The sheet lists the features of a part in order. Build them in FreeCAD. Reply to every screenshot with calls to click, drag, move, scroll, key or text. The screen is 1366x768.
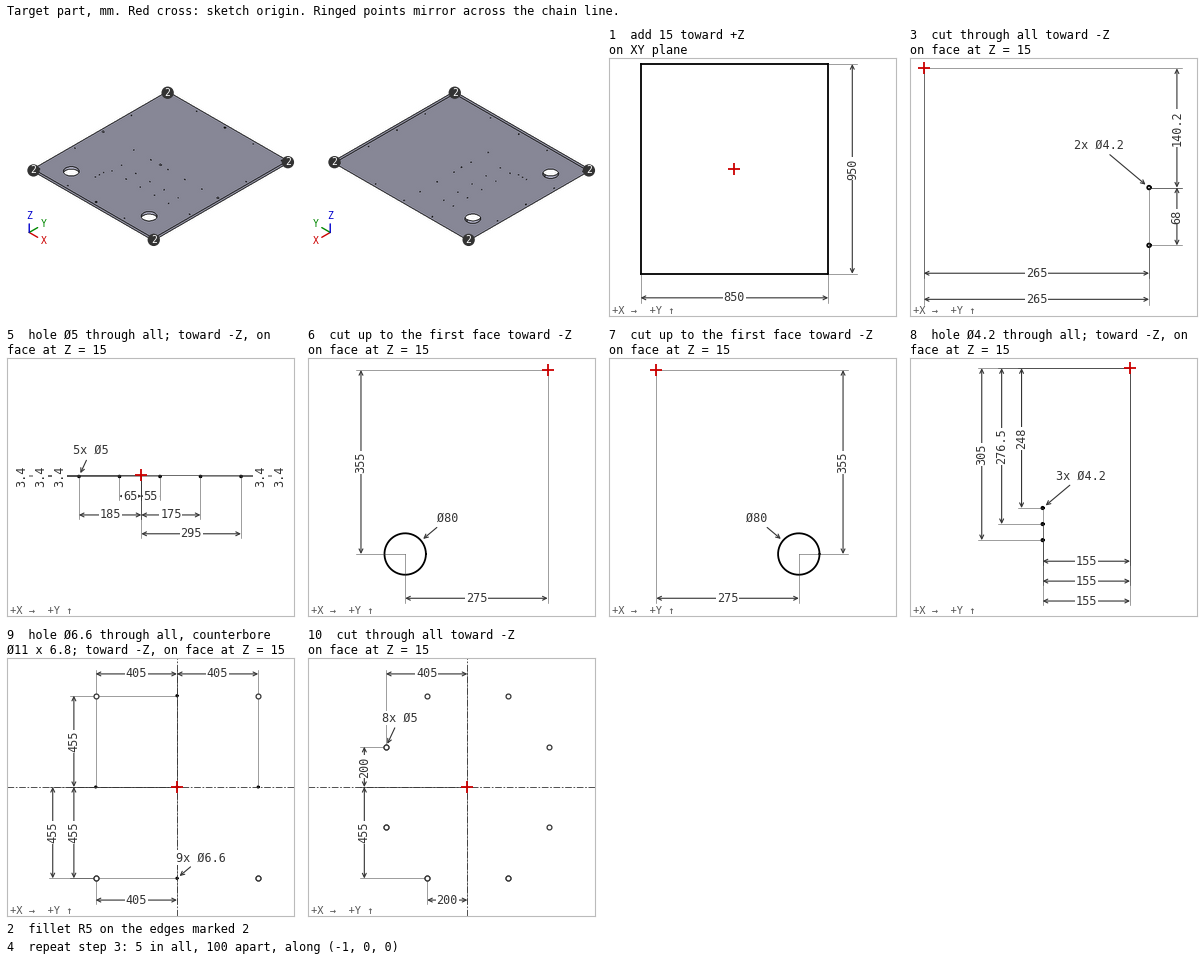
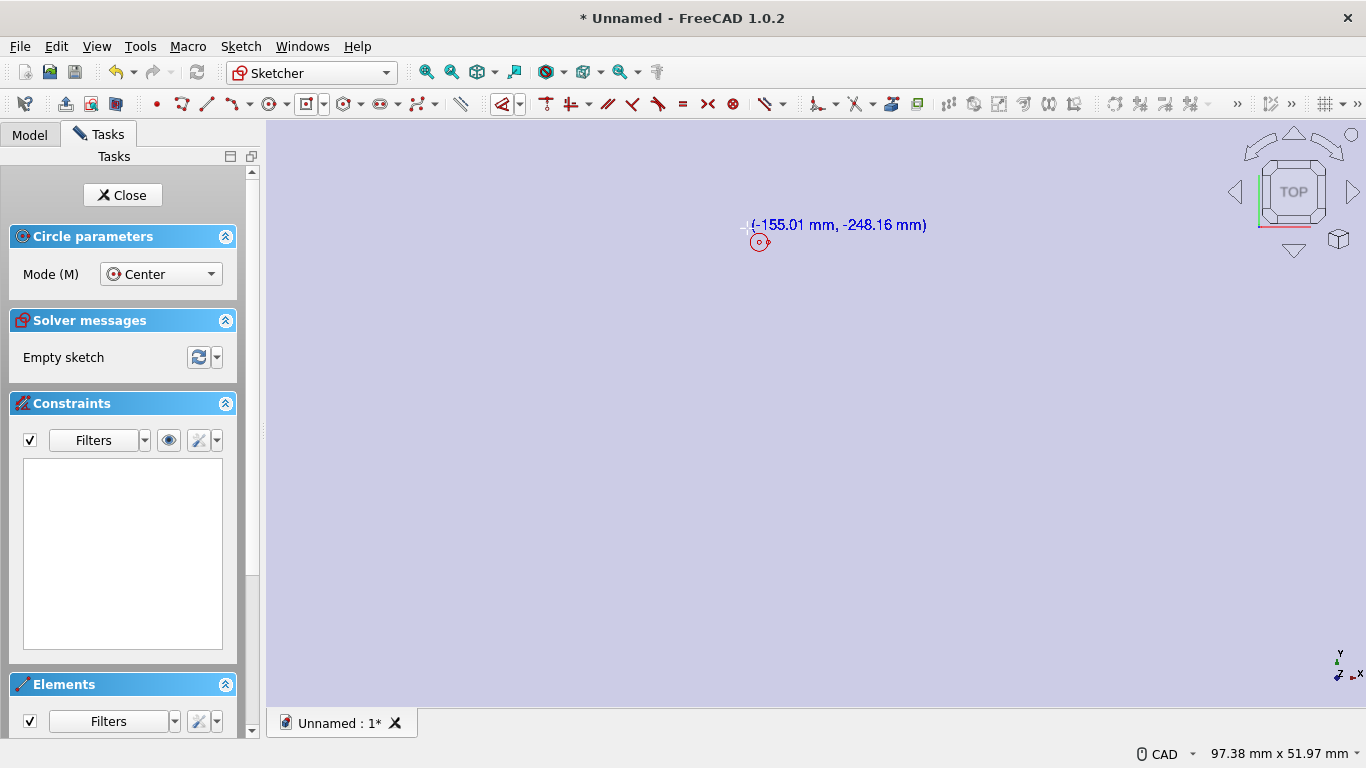
click(747, 228)
move(764, 211)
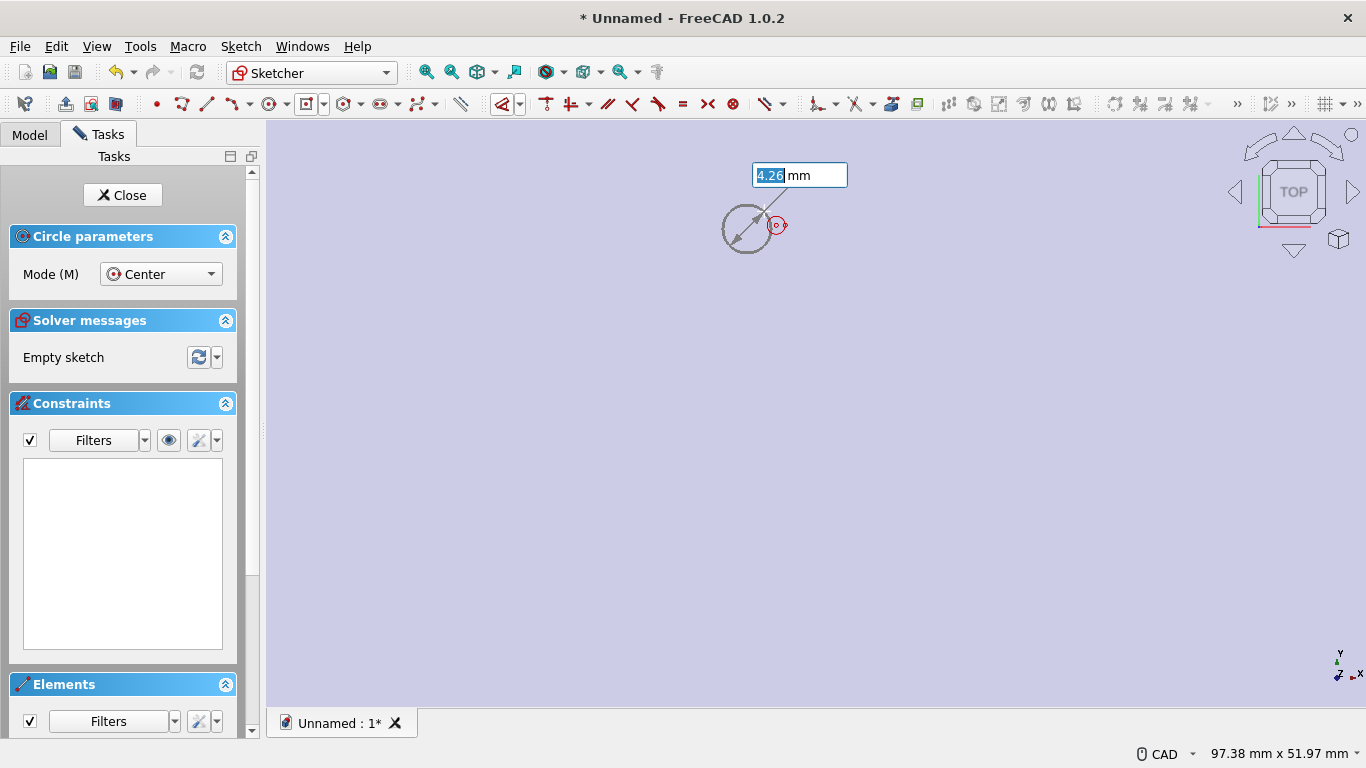
text(4.2)
key(Return)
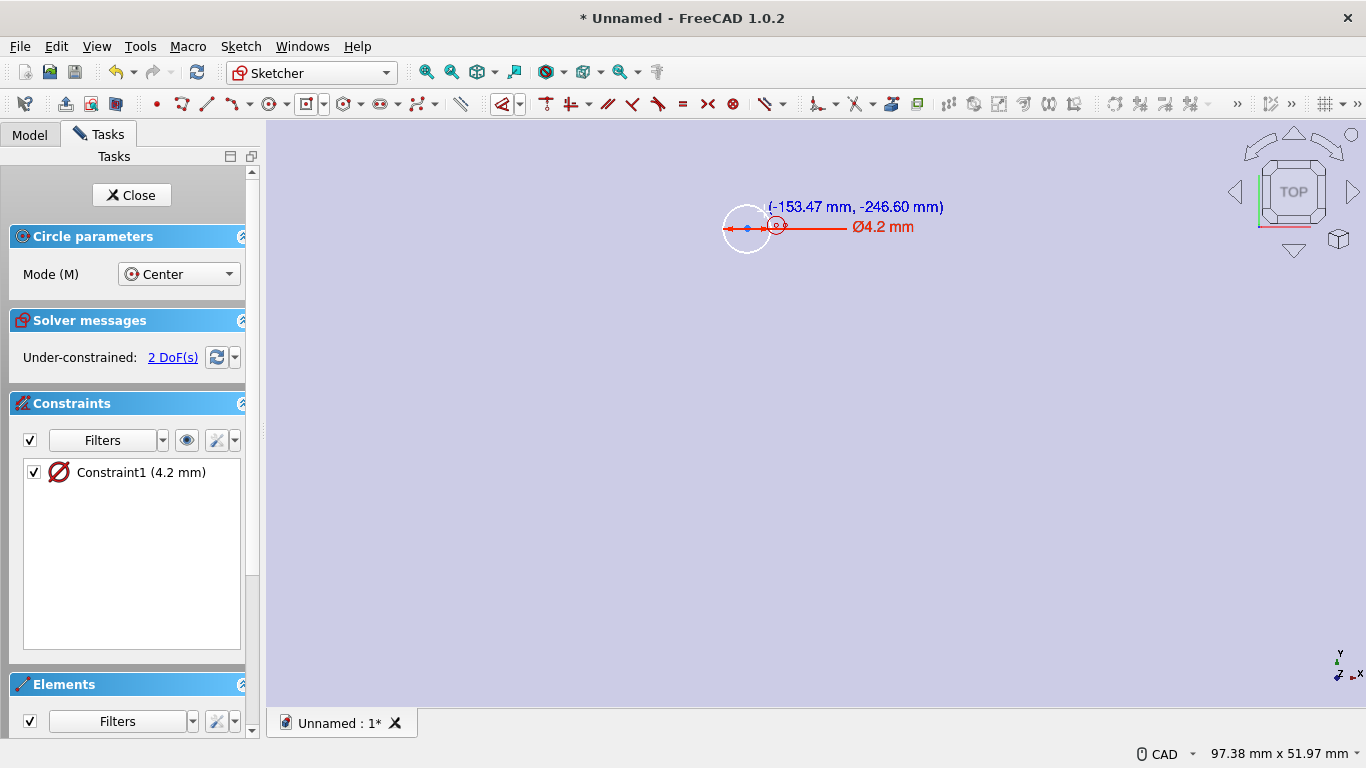
click(747, 550)
move(764, 533)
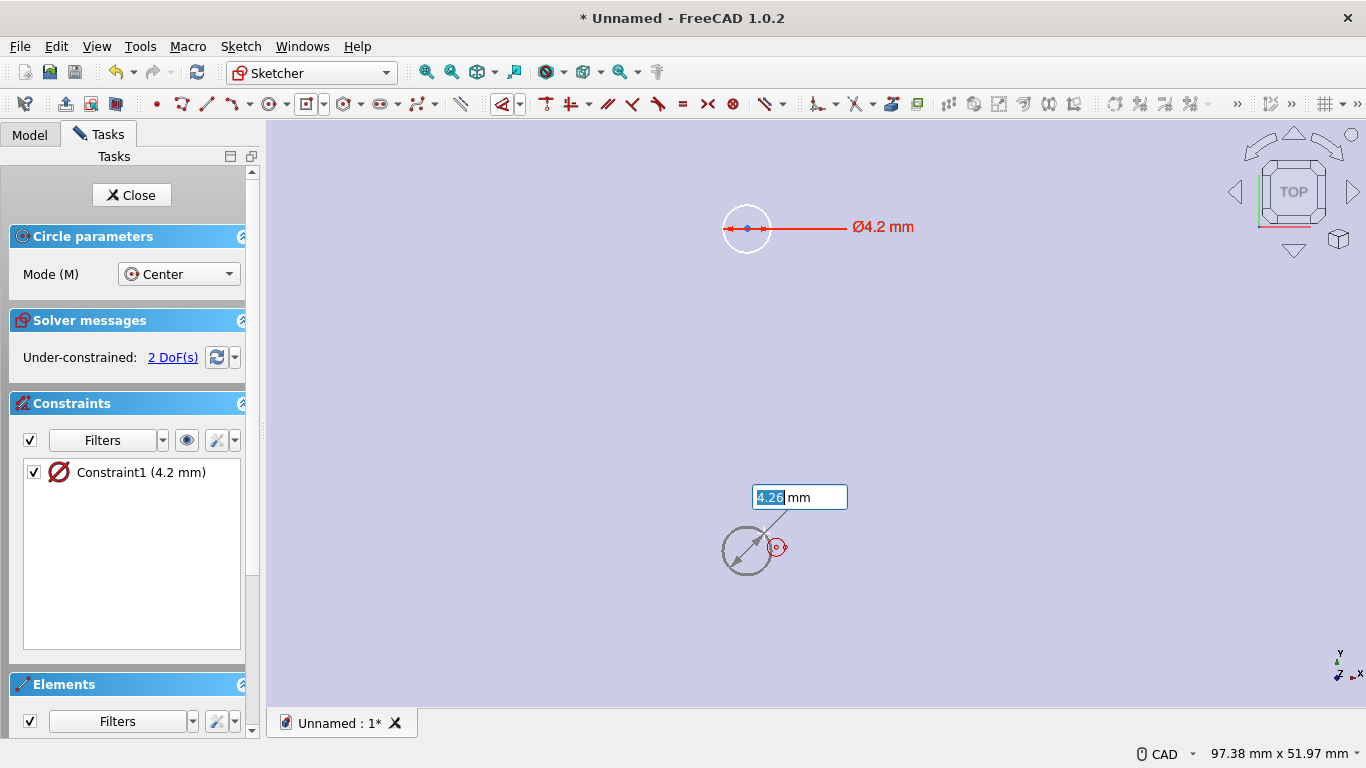
text(4.2)
key(Return)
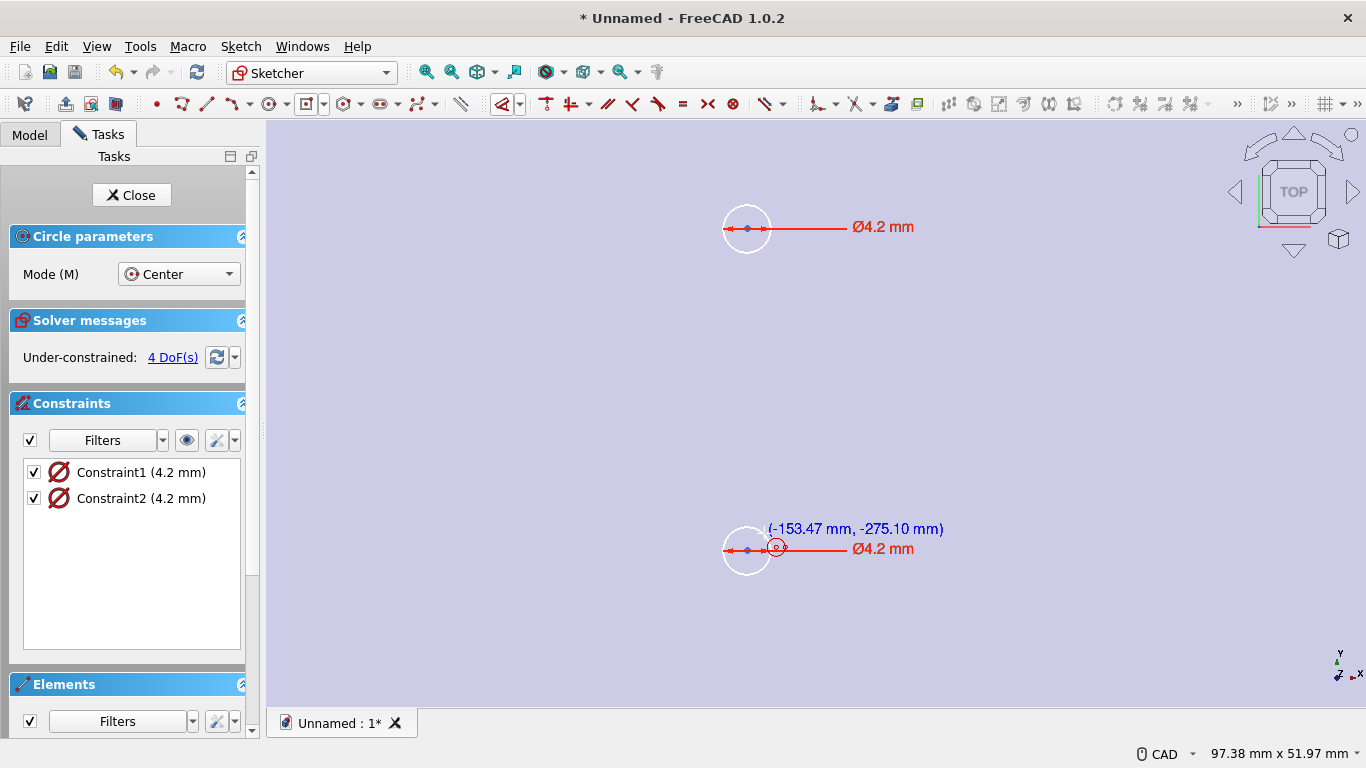
scroll(748, 248, down, 3)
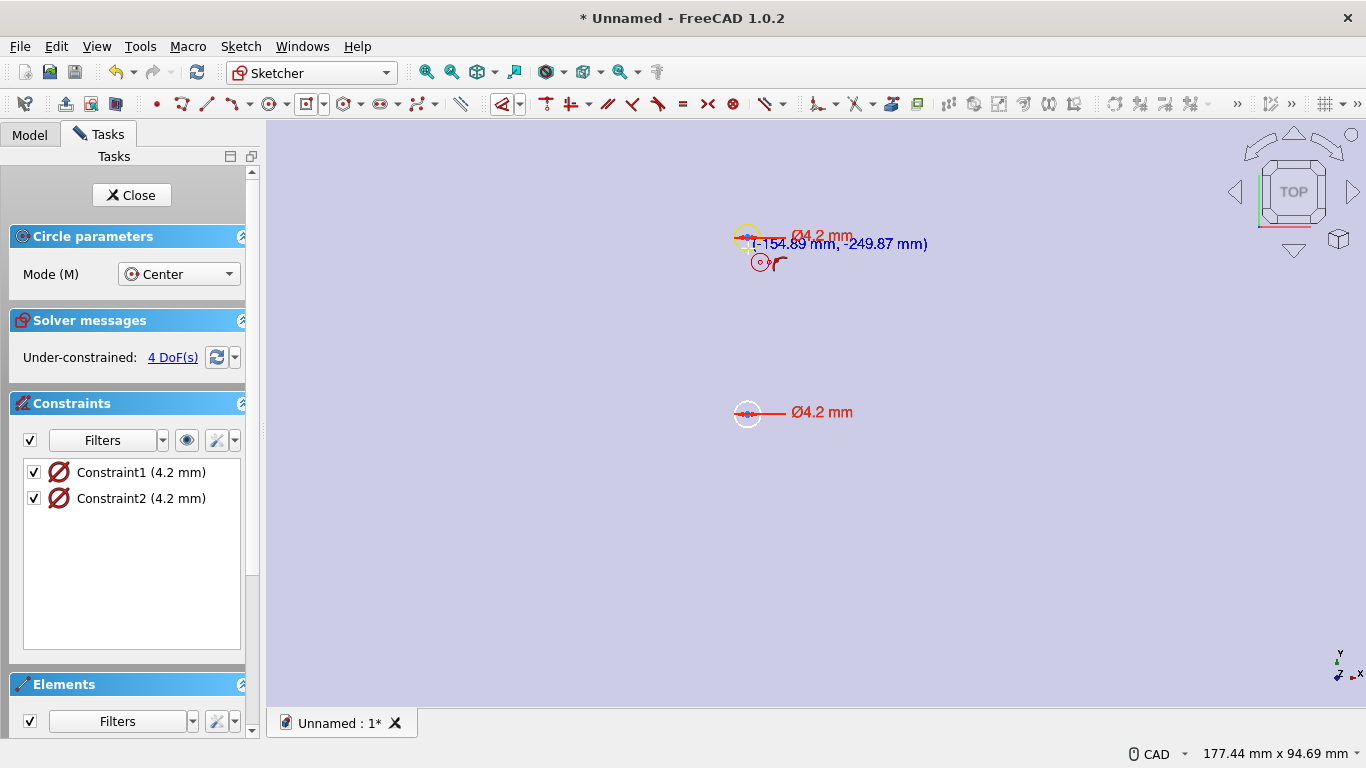
scroll(748, 590, up, 3)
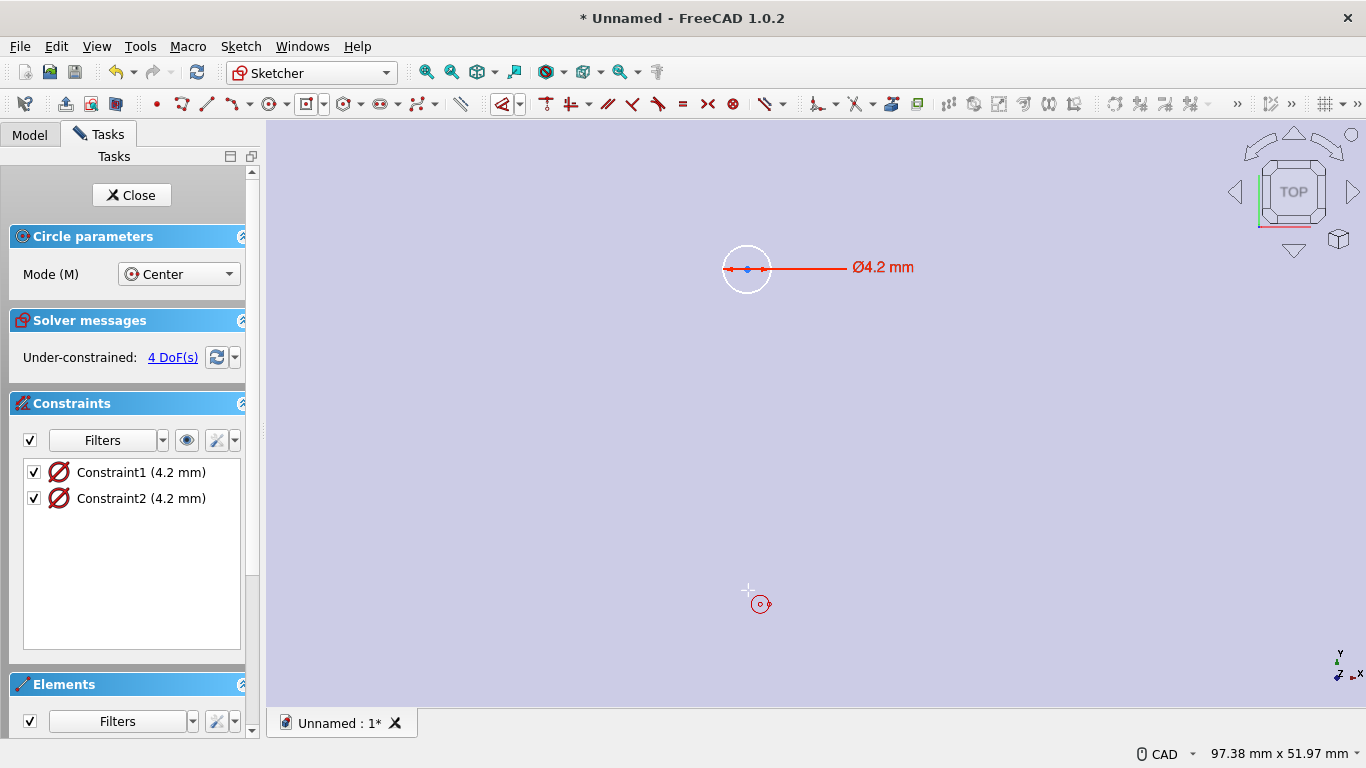
click(747, 590)
move(764, 573)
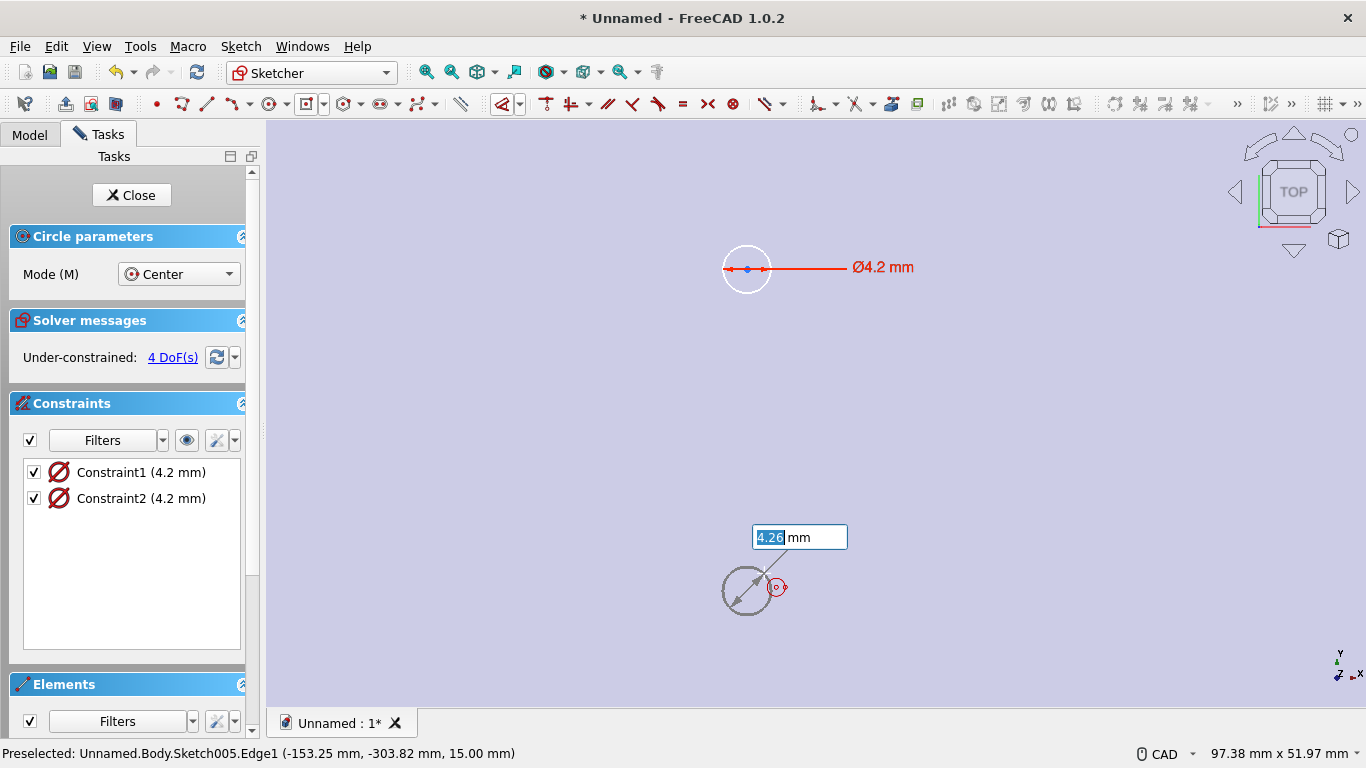
text(4.2)
key(Return)
key(Escape)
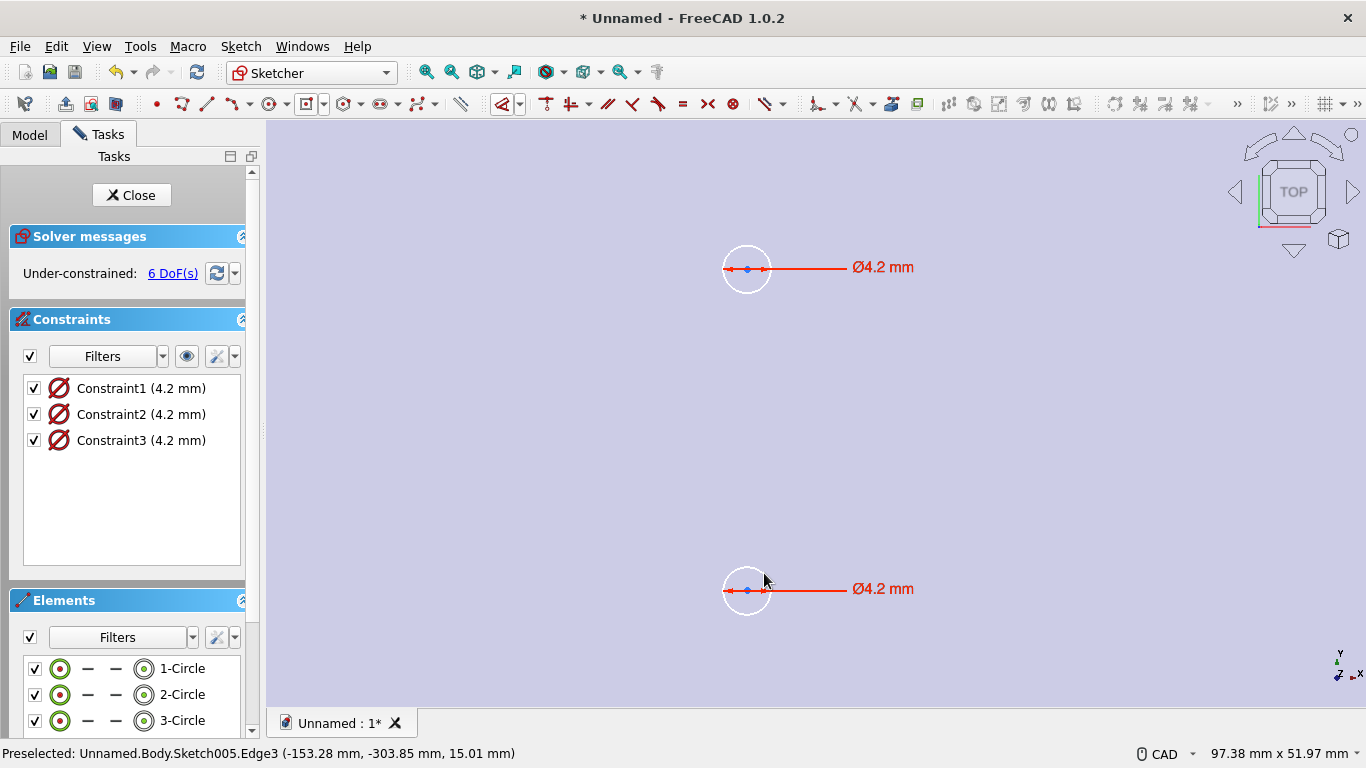
scroll(748, 590, down, 3)